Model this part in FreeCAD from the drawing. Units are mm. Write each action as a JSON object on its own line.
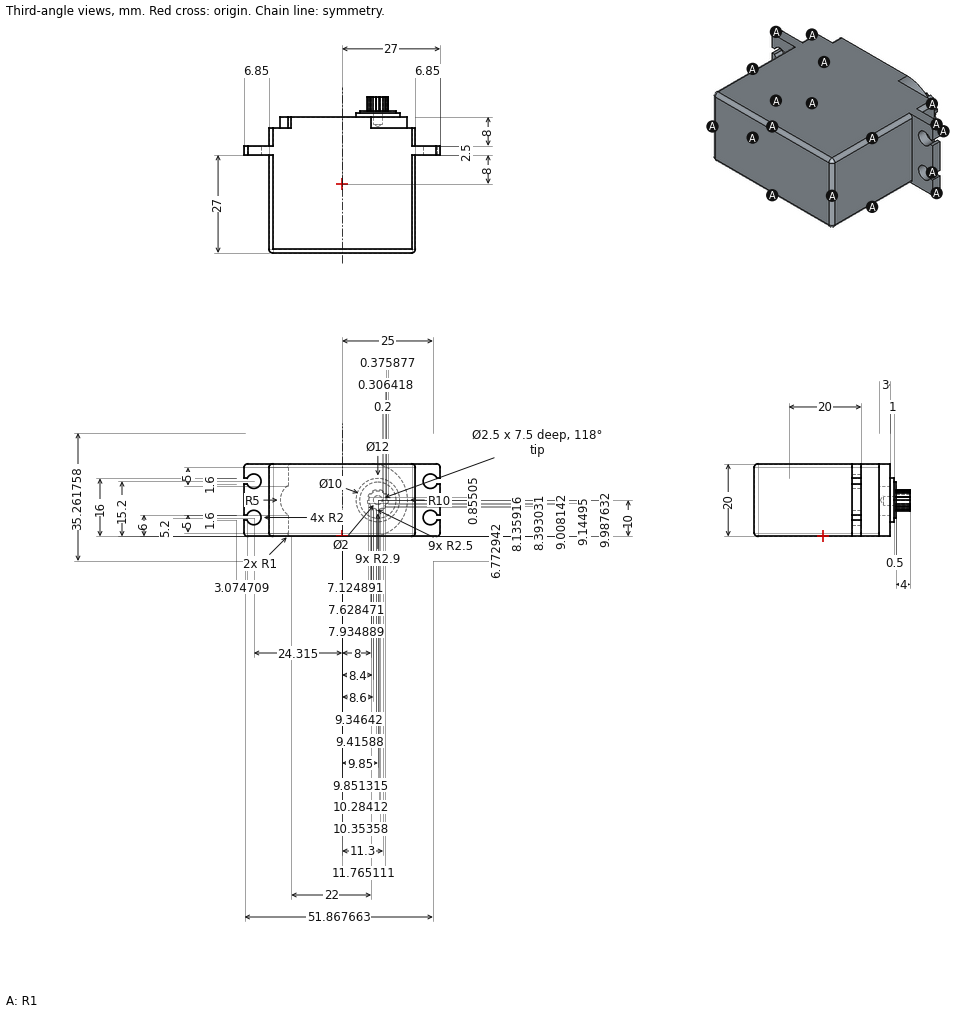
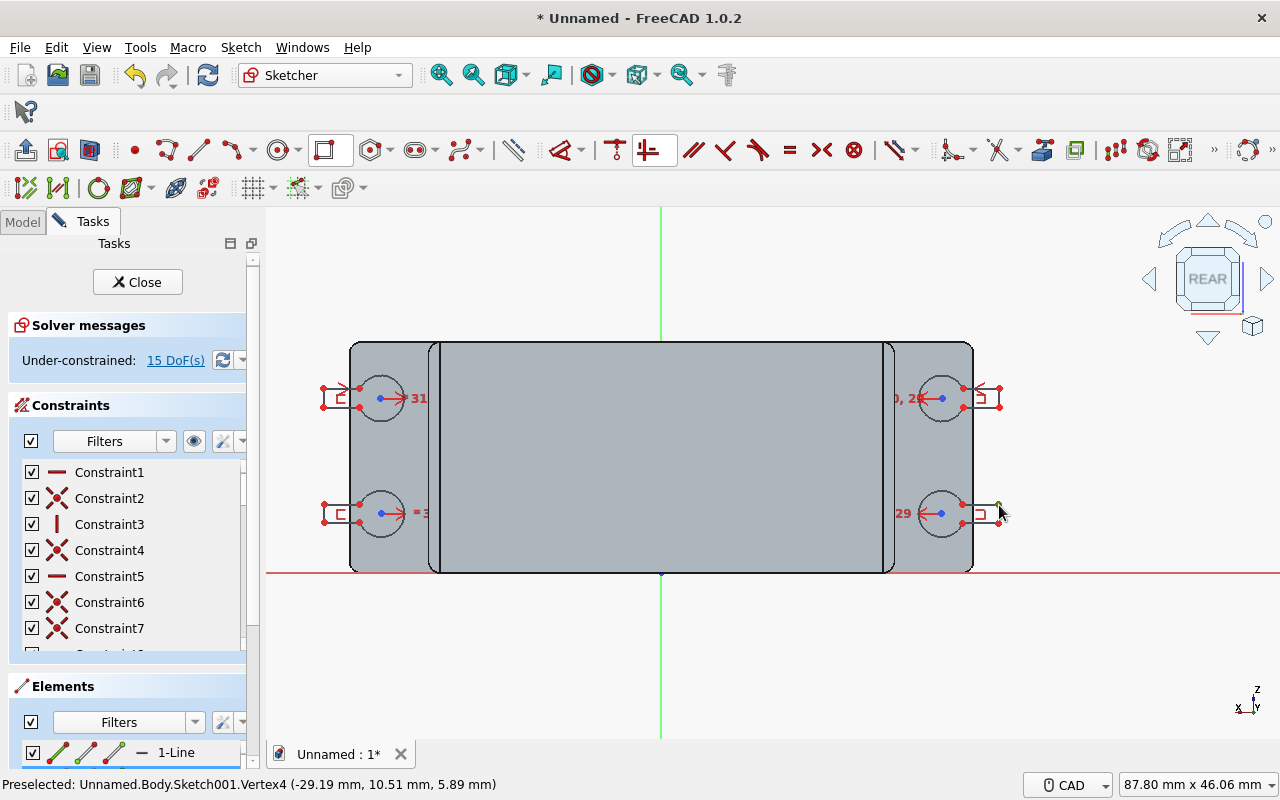
{"action": "left_click", "coordinate": [324, 505]}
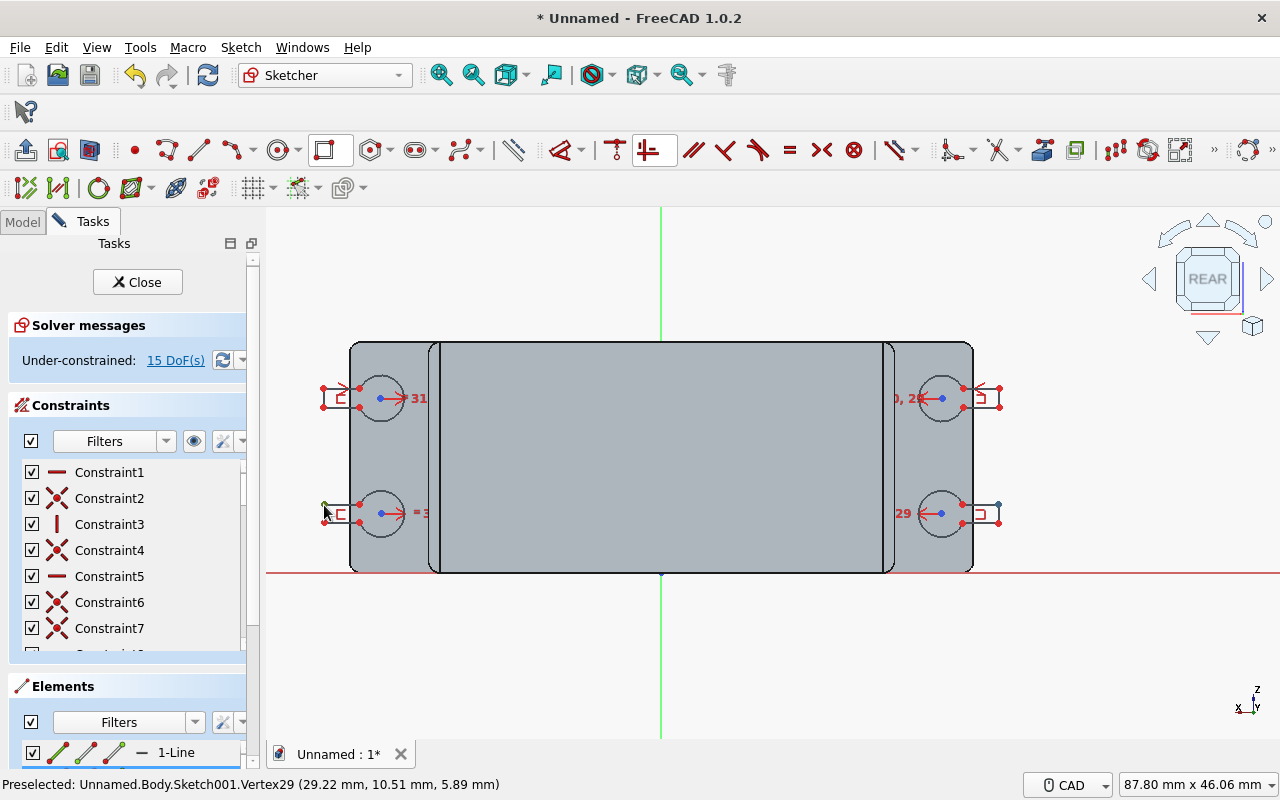
{"action": "left_click", "coordinate": [661, 677]}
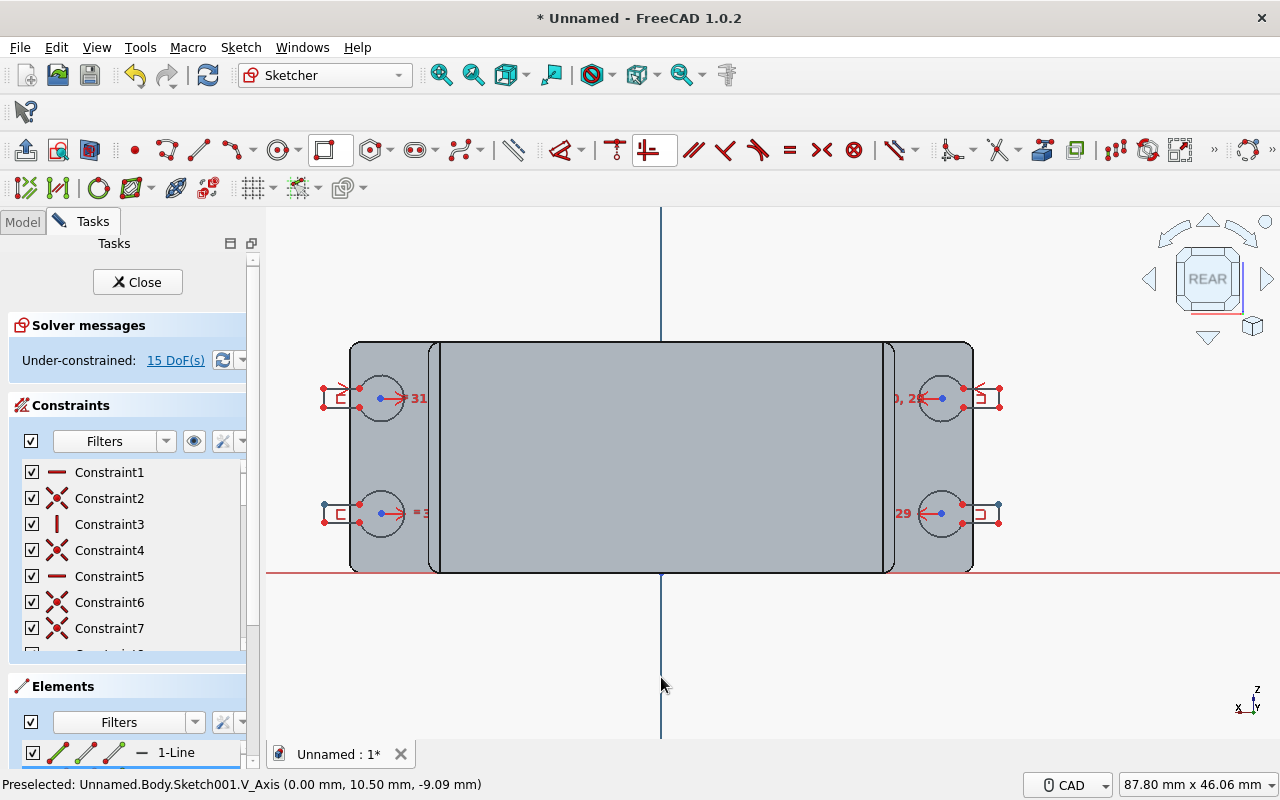
{"action": "left_click", "coordinate": [822, 150]}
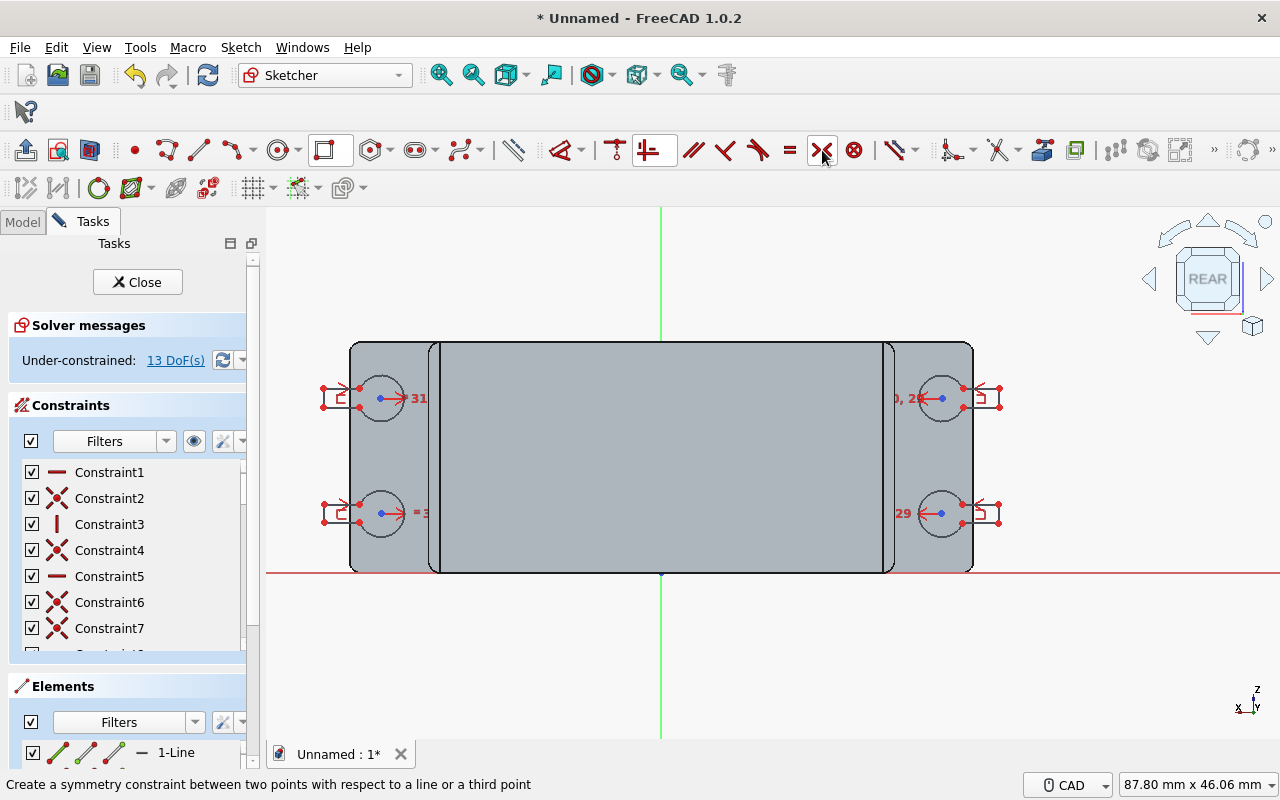
{"action": "left_click", "coordinate": [560, 150]}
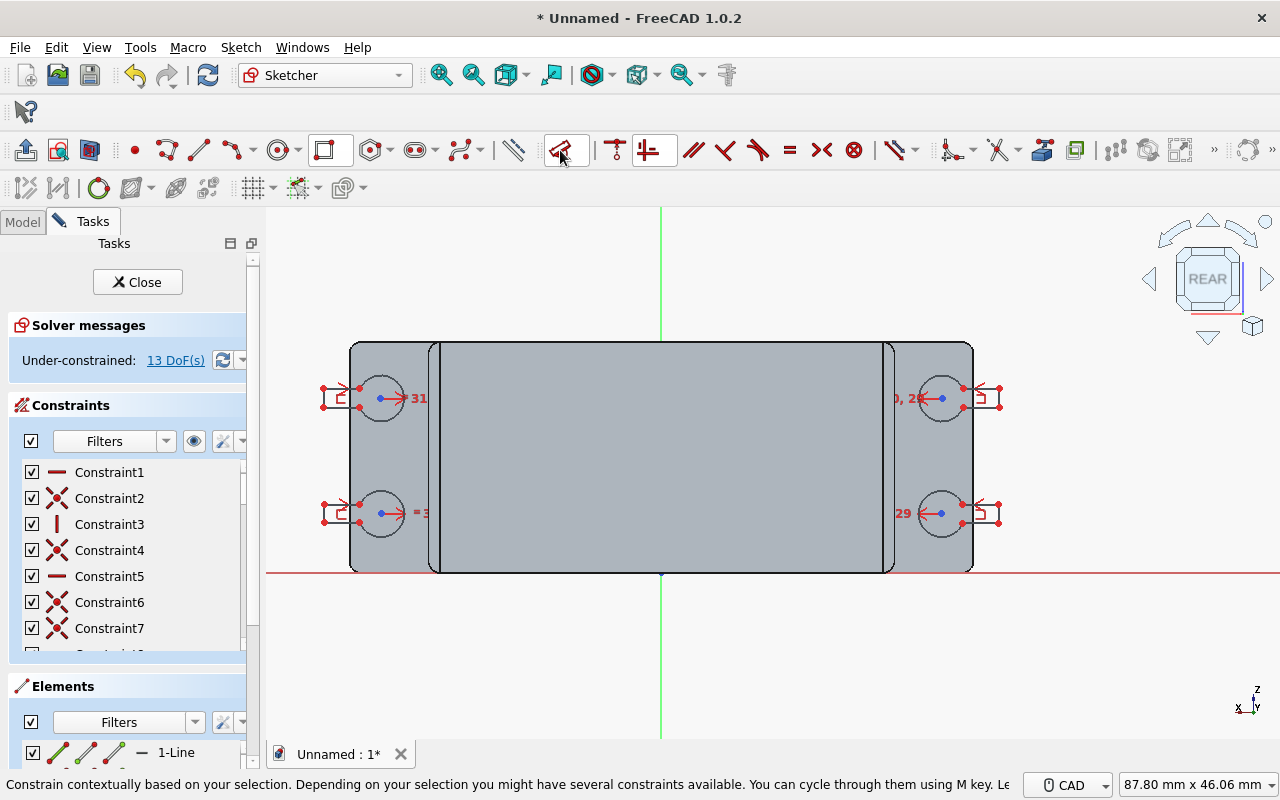
{"action": "scroll", "coordinate": [931, 494], "scroll_direction": "up", "scroll_amount": 3}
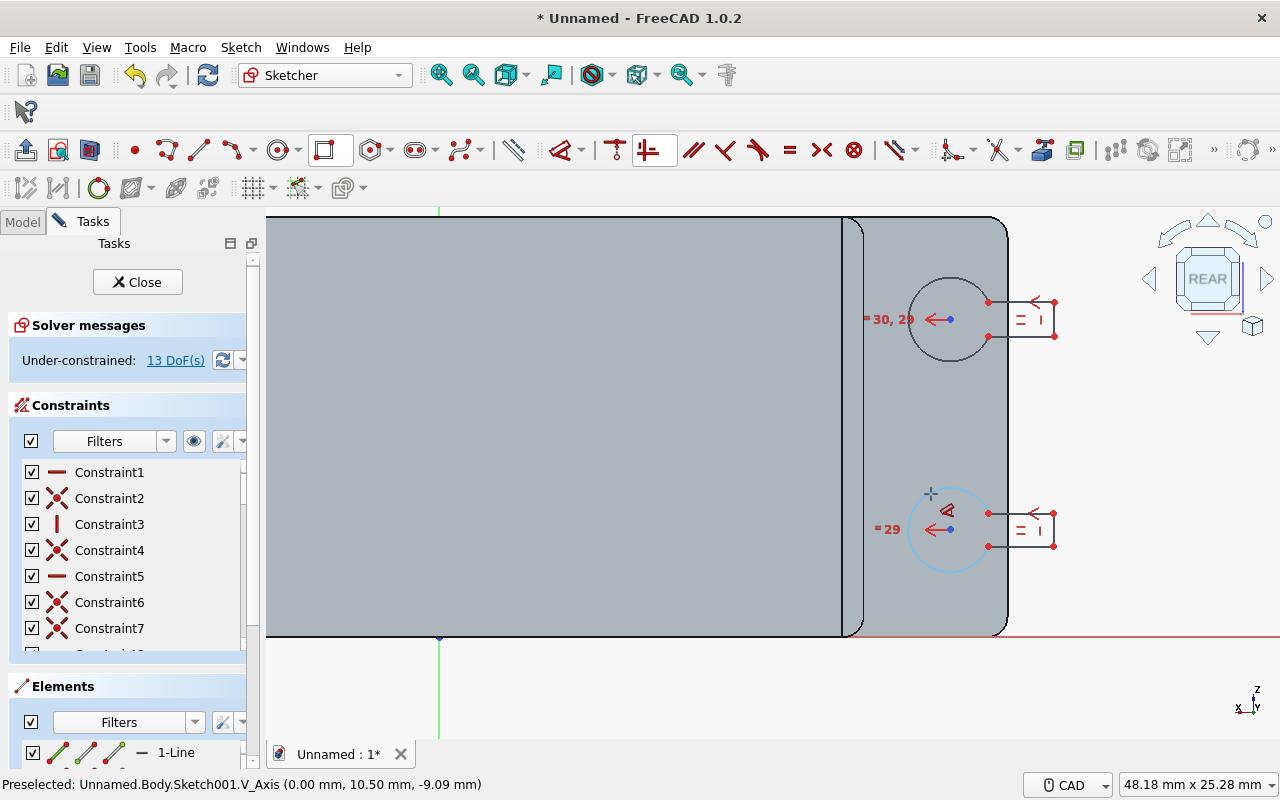
{"action": "left_click", "coordinate": [931, 493]}
{"action": "left_click", "coordinate": [916, 465]}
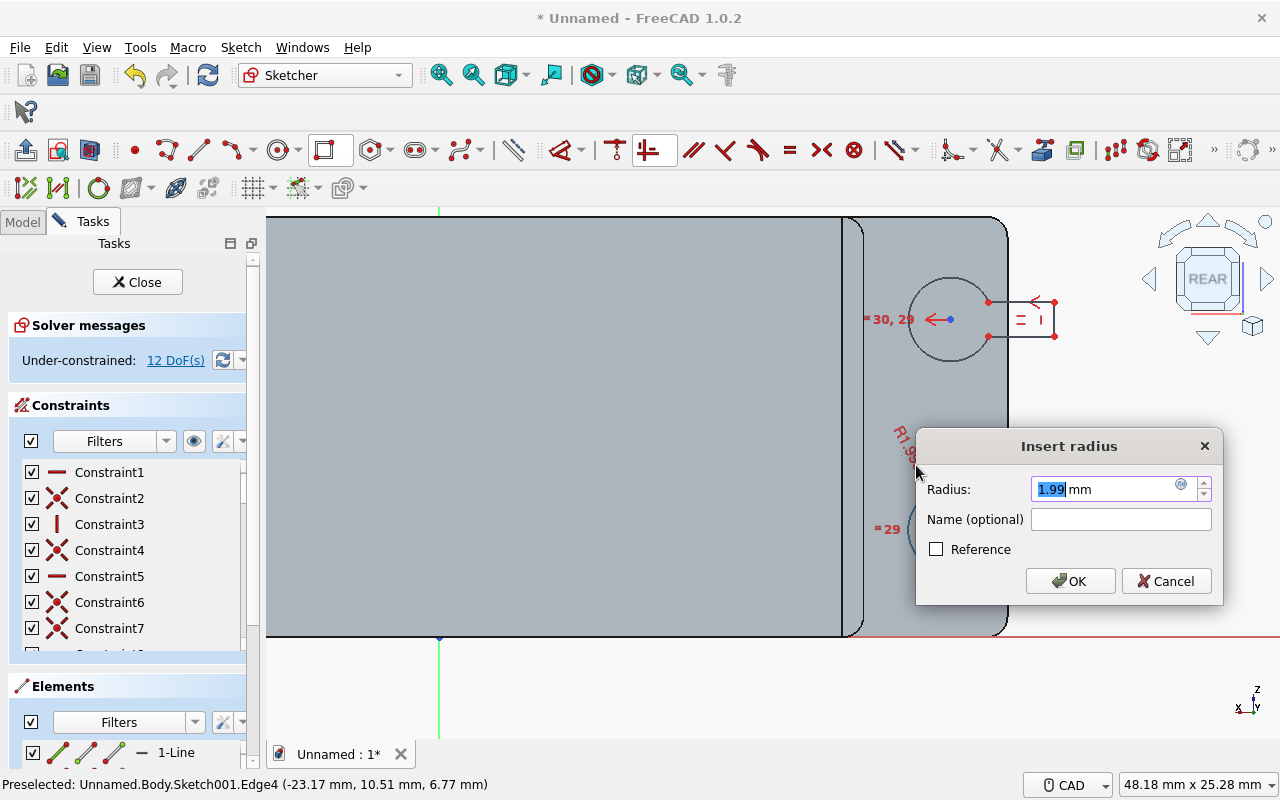
{"action": "type", "text": "2"}
{"action": "key", "text": "Return"}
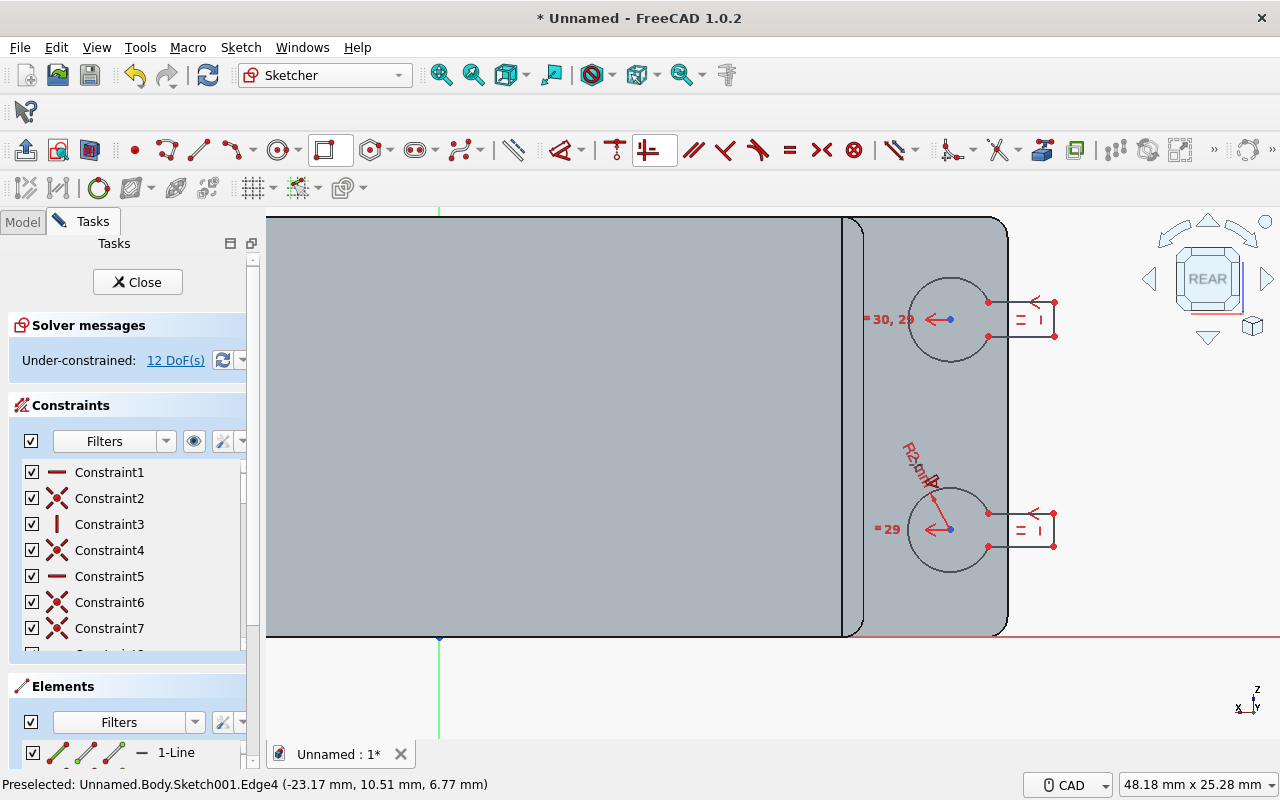
{"action": "left_click", "coordinate": [1054, 514]}
{"action": "left_click", "coordinate": [1088, 576]}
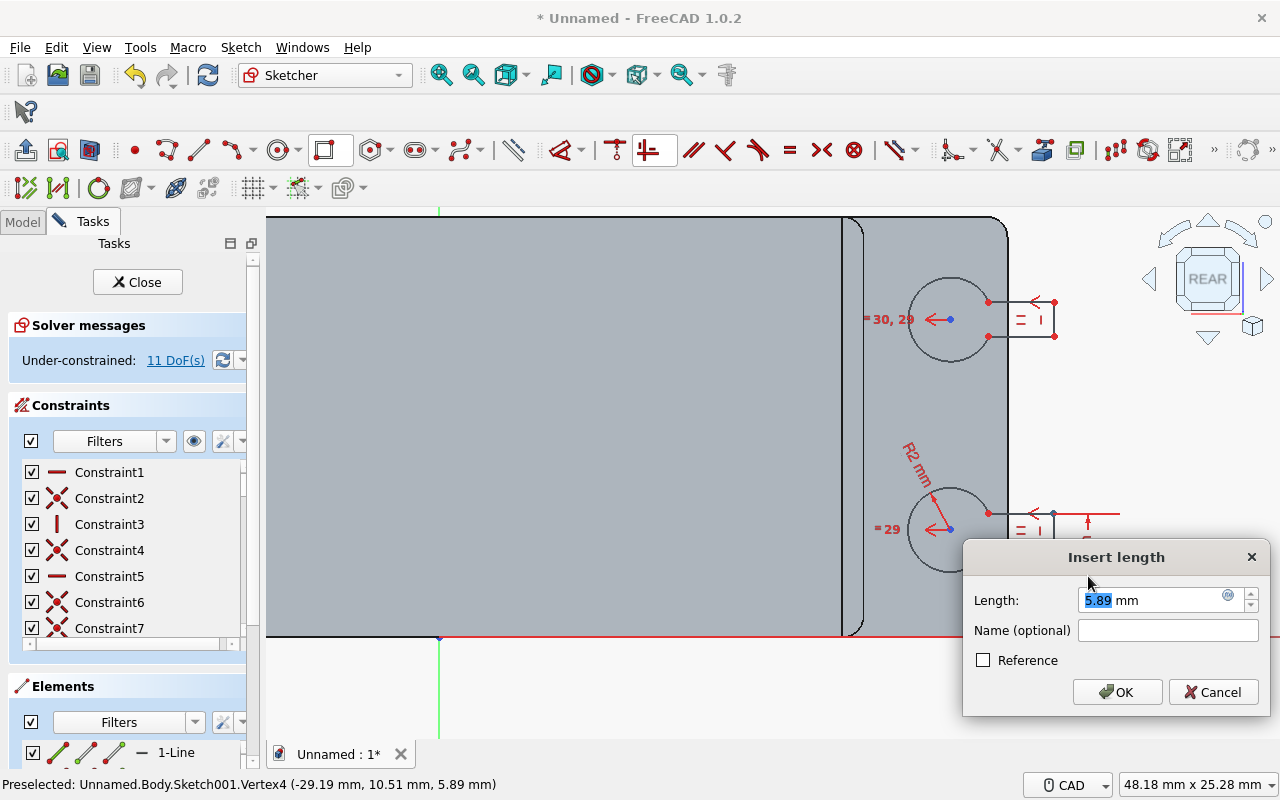
{"action": "type", "text": "6"}
{"action": "key", "text": "Return"}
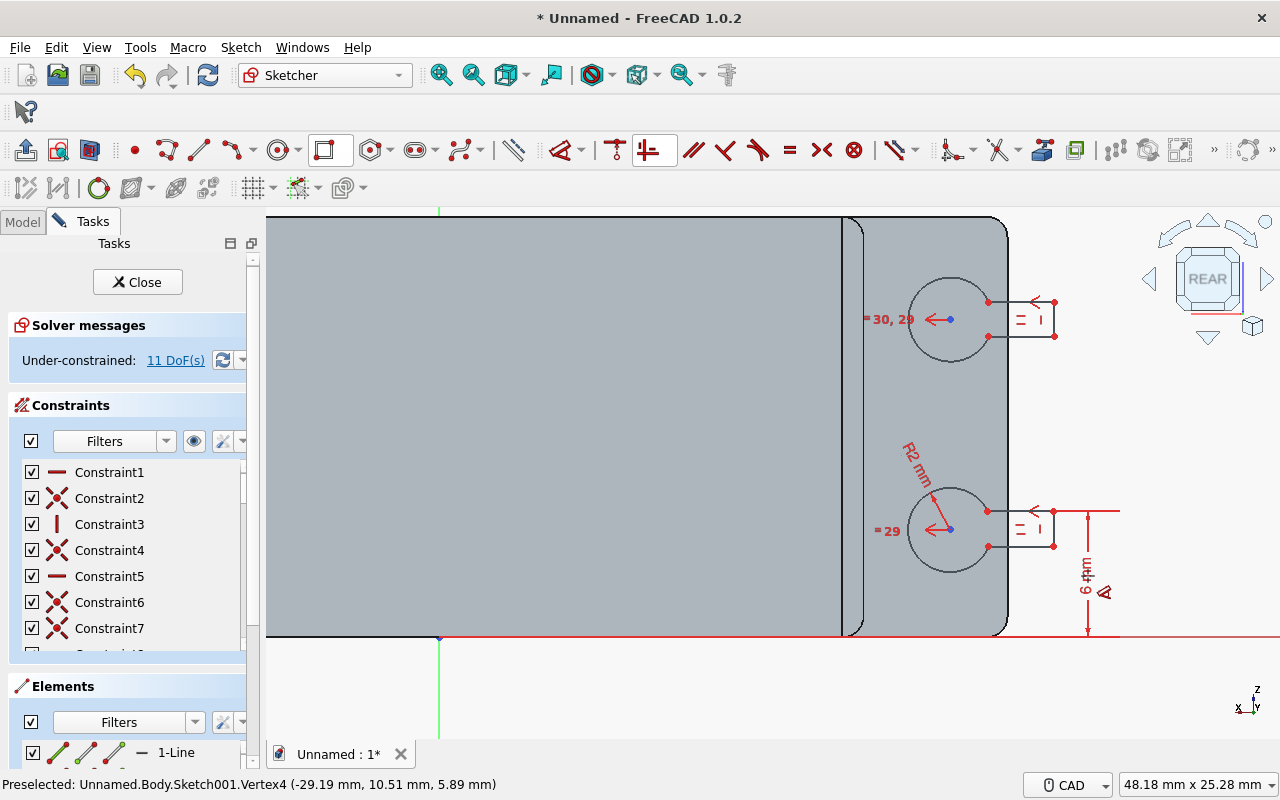
{"action": "scroll", "coordinate": [1054, 536], "scroll_direction": "up", "scroll_amount": 2}